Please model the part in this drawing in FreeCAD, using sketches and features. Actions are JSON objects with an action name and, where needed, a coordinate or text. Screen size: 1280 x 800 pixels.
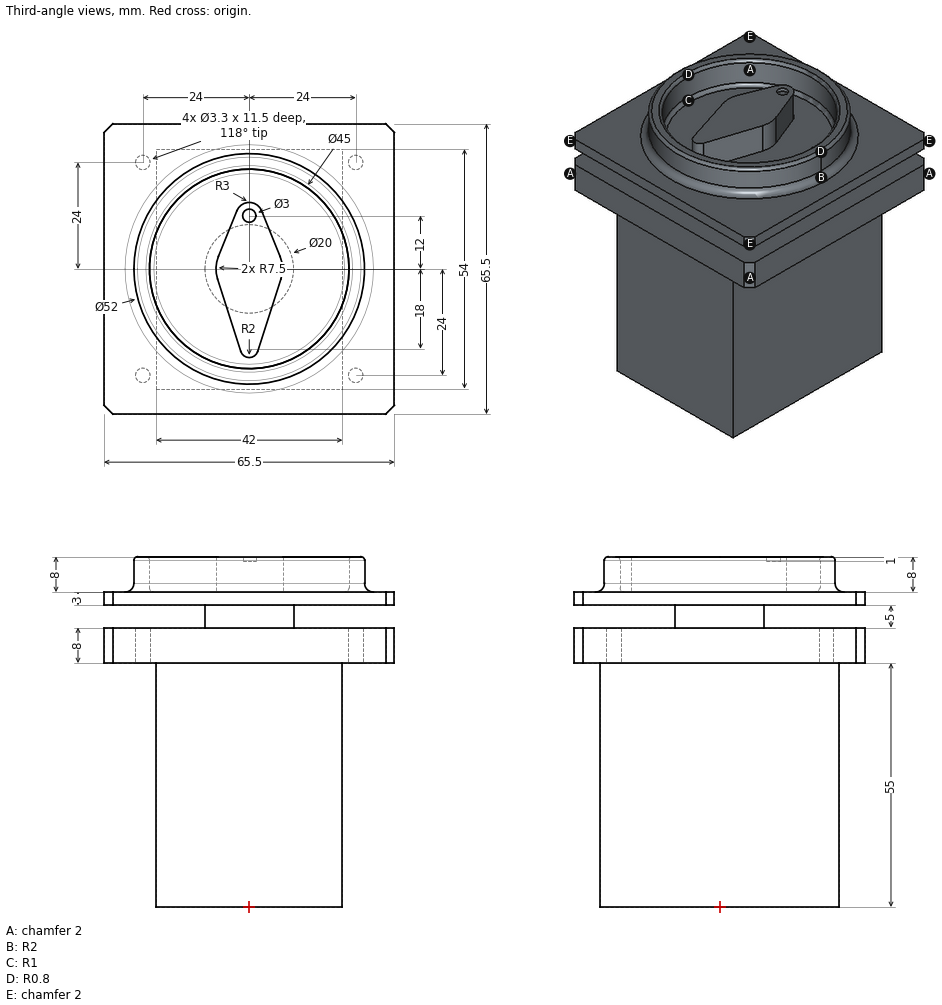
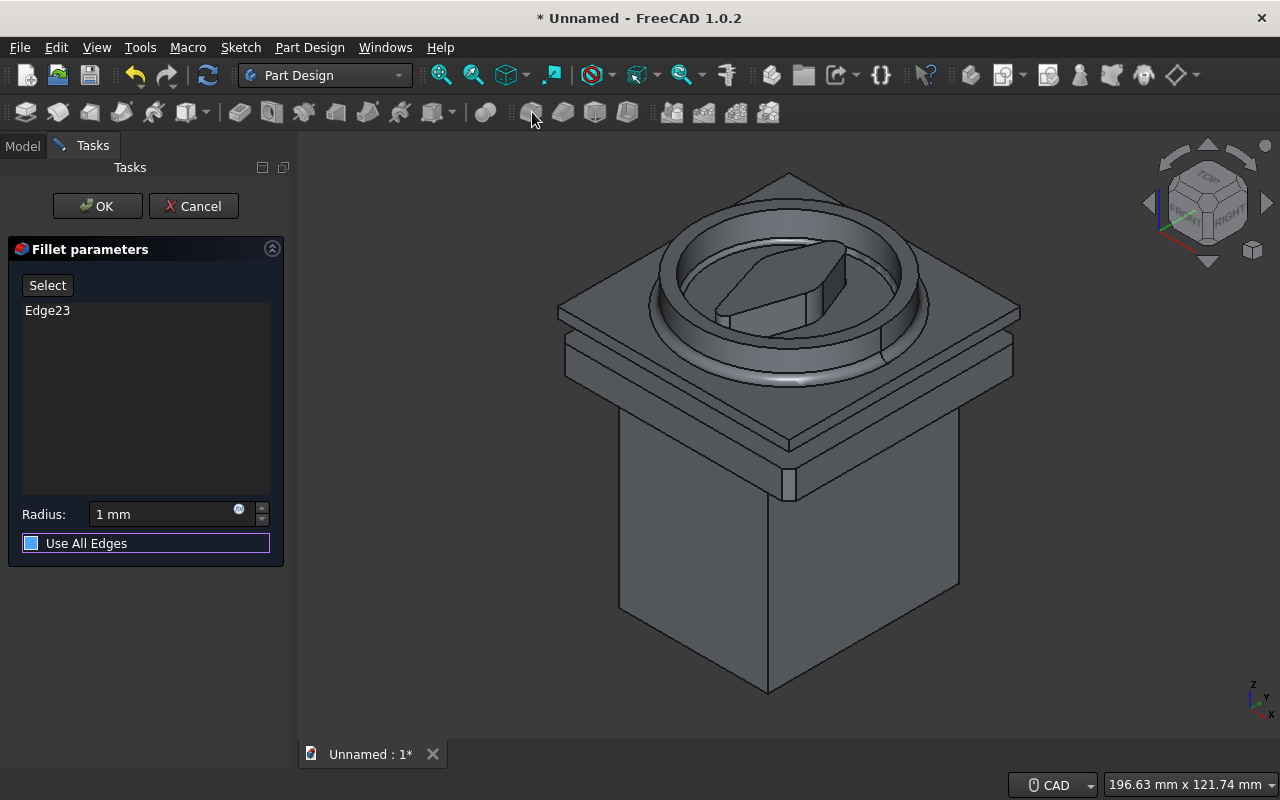
{"action": "left_click", "coordinate": [98, 206]}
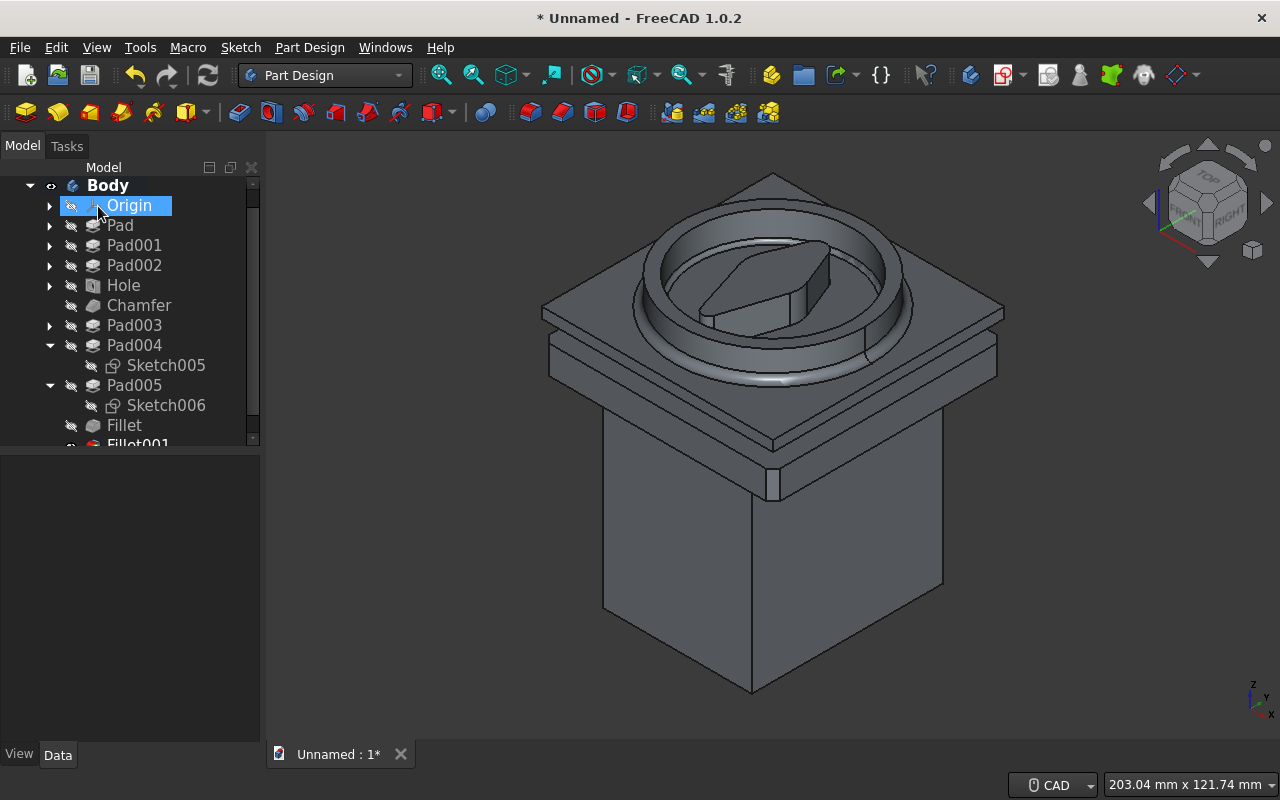
{"action": "left_click", "coordinate": [657, 307]}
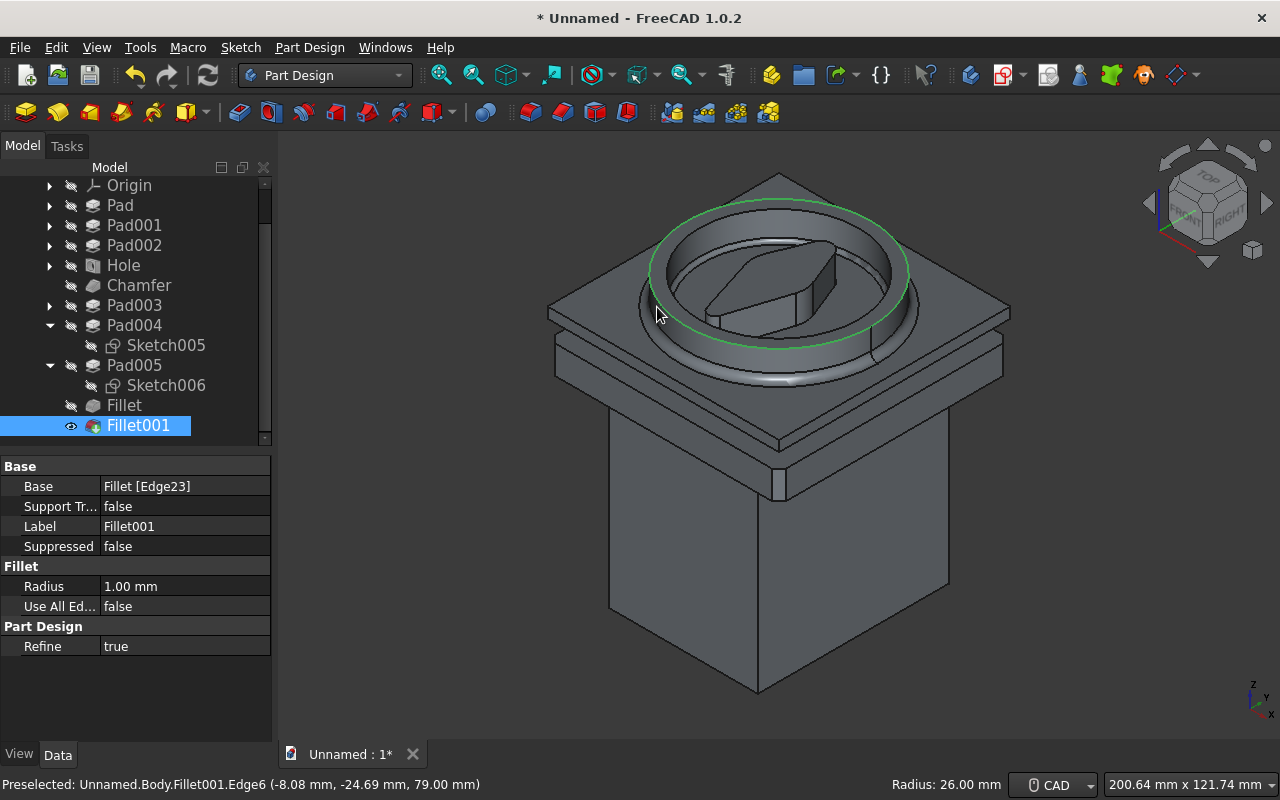
{"action": "left_click", "coordinate": [700, 227], "text": "ctrl"}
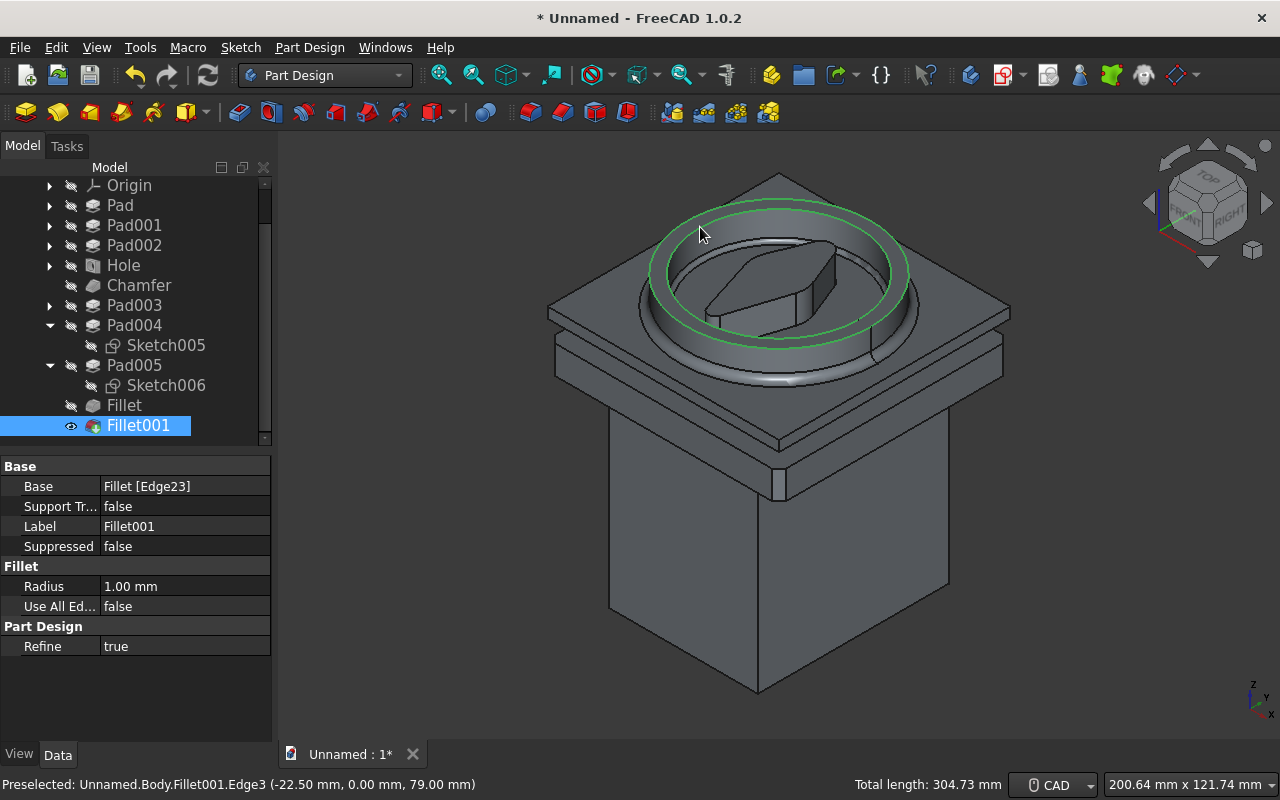
{"action": "left_click", "coordinate": [532, 112]}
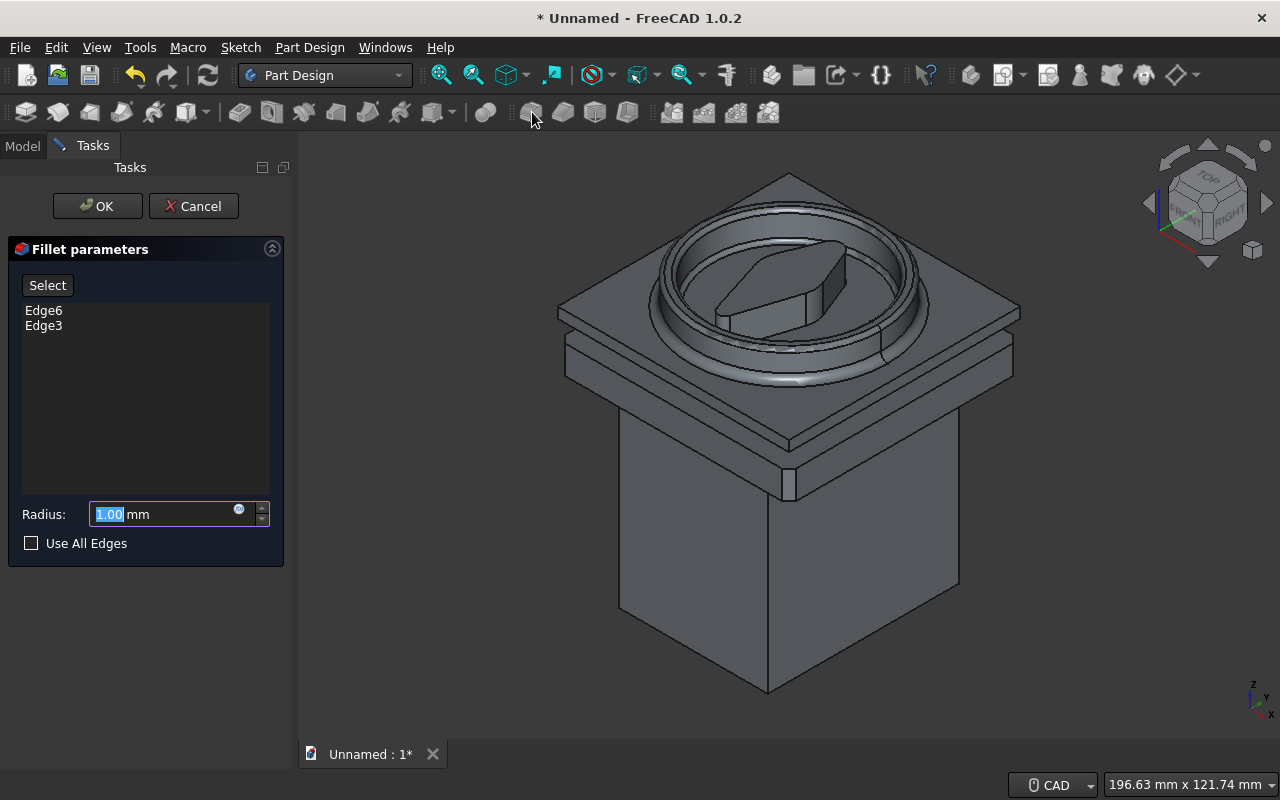
{"action": "type", "text": "0.8"}
{"action": "key", "text": "Tab"}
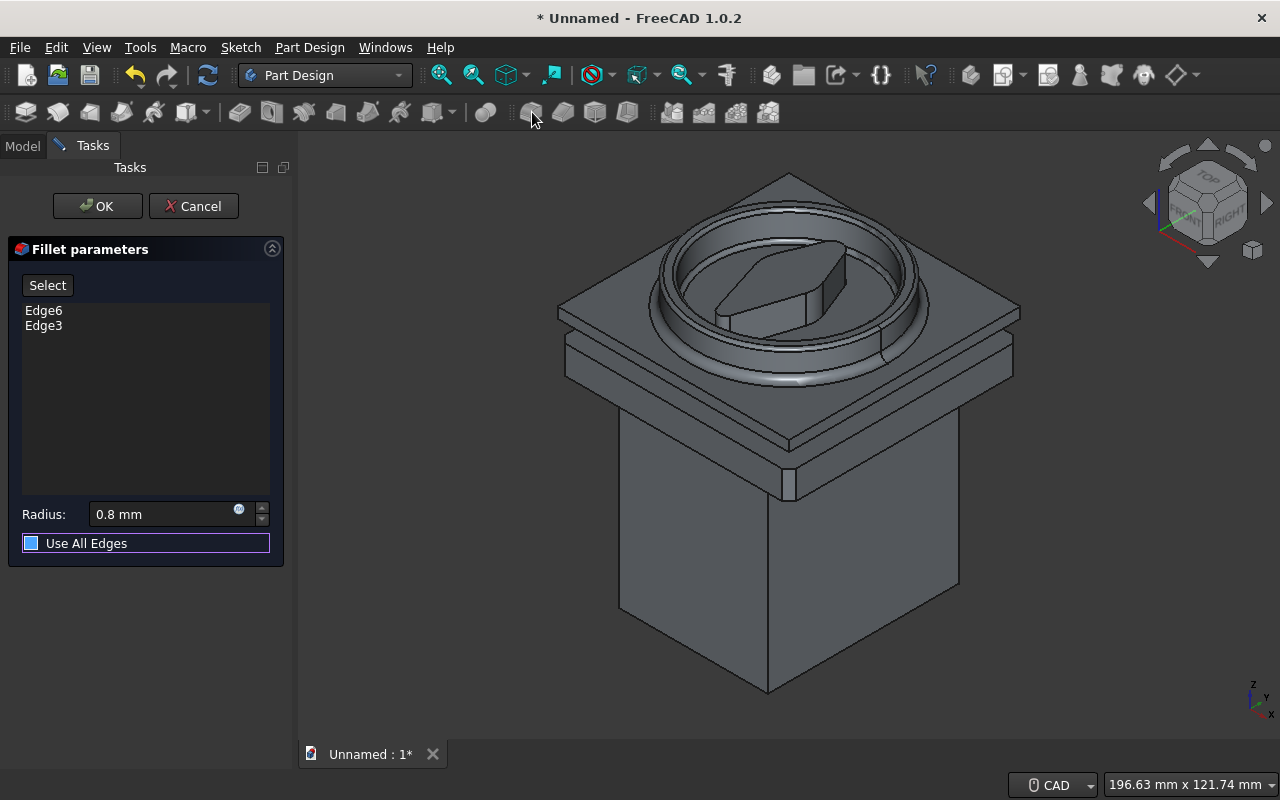
{"action": "left_click", "coordinate": [98, 206]}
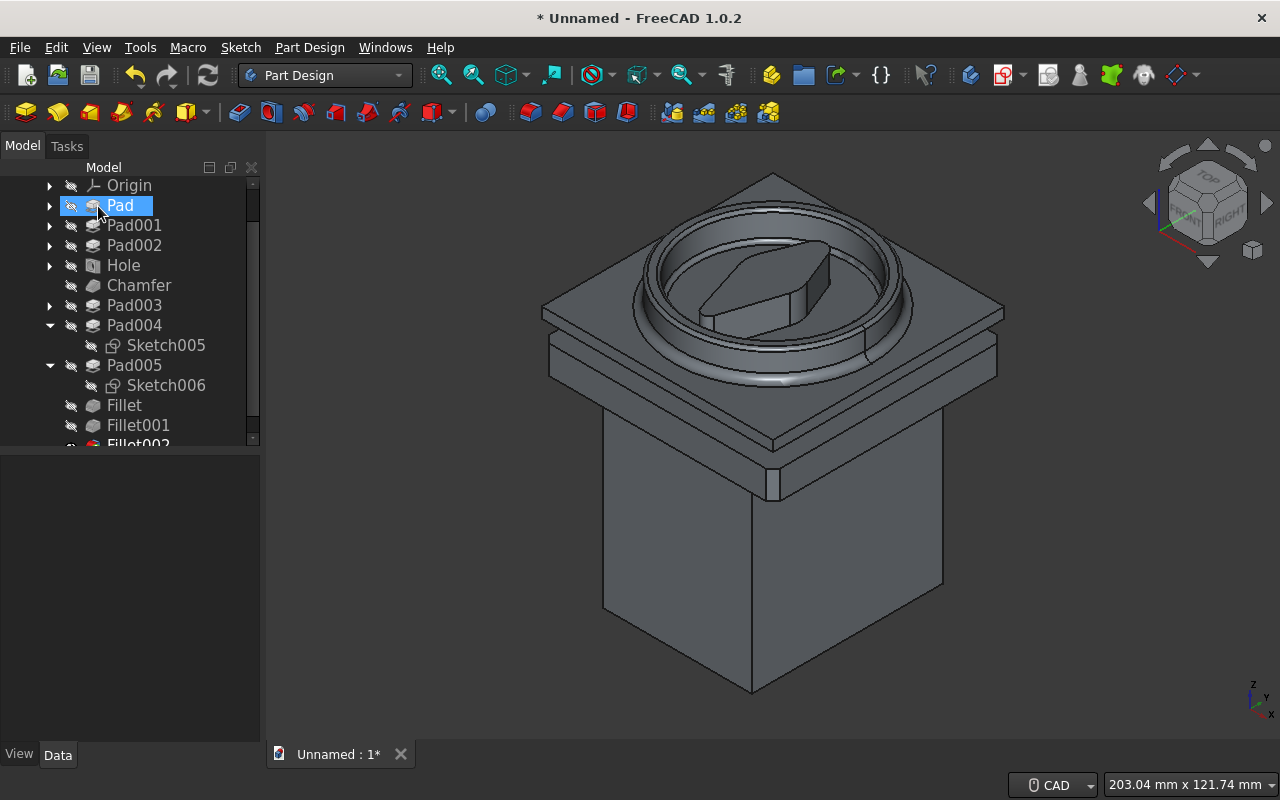
{"action": "left_click", "coordinate": [764, 278]}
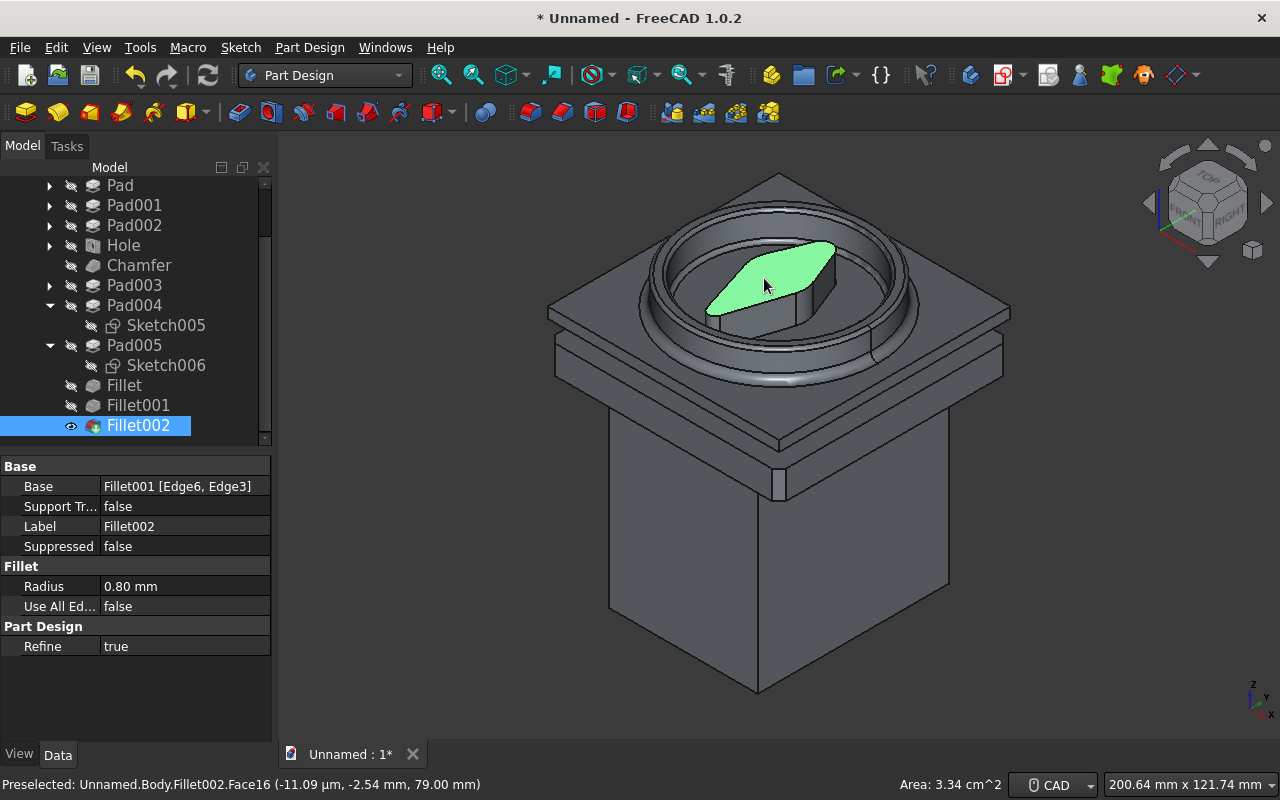
{"action": "left_click", "coordinate": [1004, 76]}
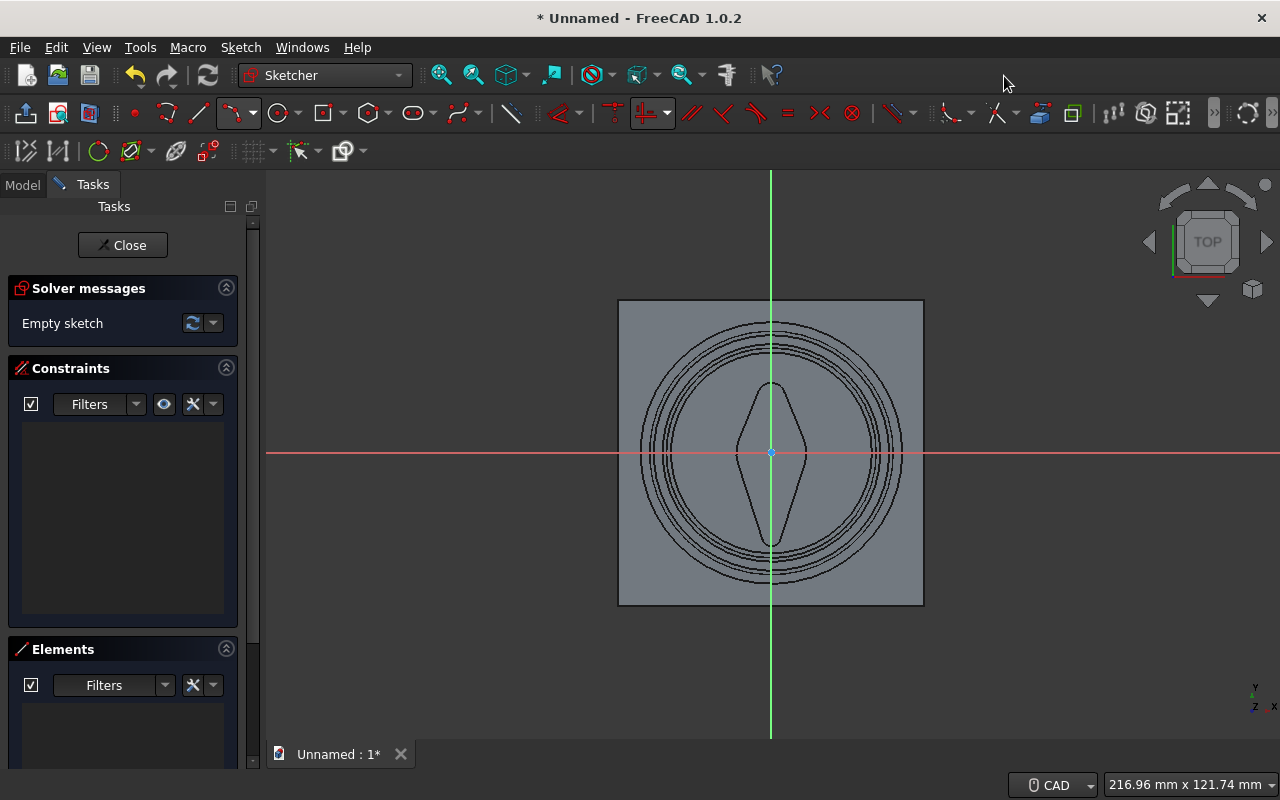
{"action": "scroll", "coordinate": [775, 394], "scroll_direction": "up", "scroll_amount": 15}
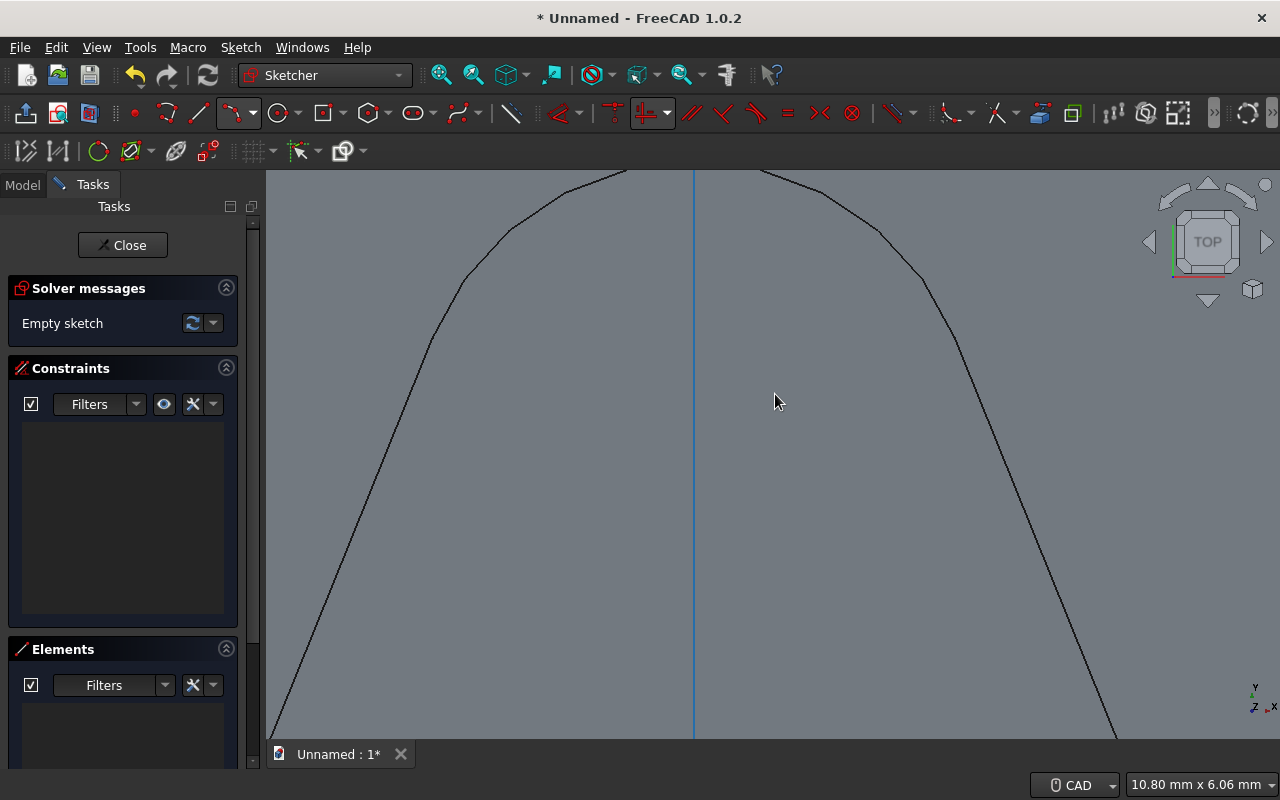
{"action": "left_click", "coordinate": [278, 114]}